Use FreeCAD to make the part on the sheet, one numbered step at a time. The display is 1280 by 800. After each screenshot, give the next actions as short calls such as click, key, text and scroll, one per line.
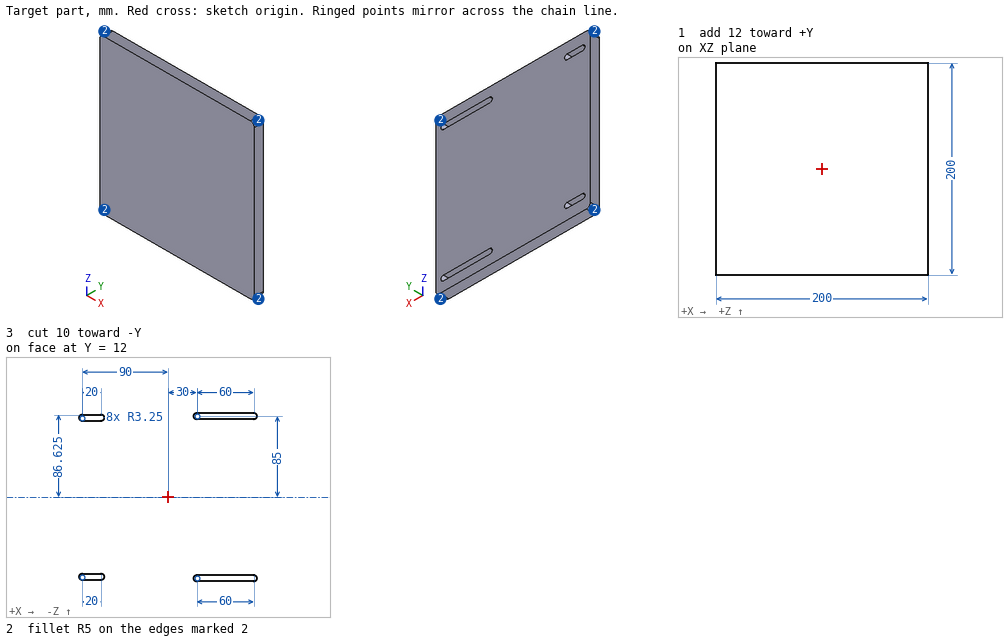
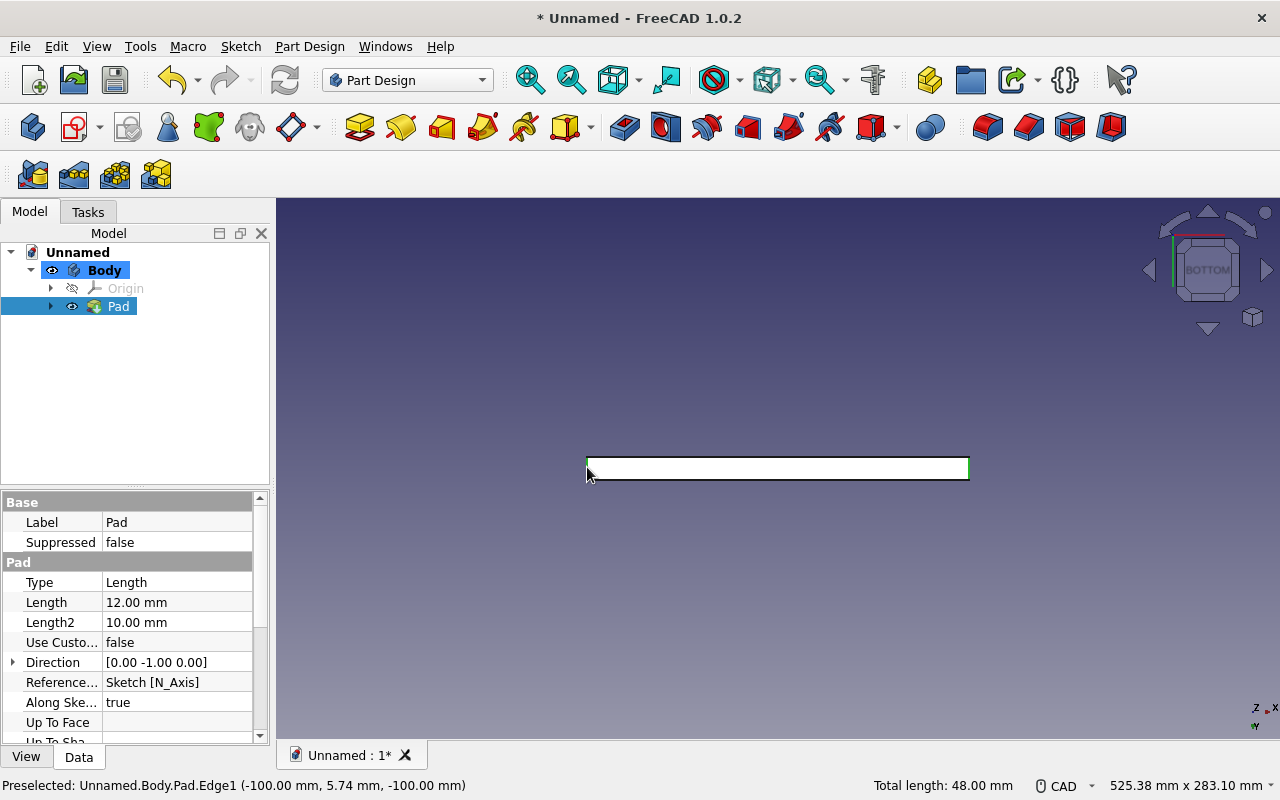
click(988, 128)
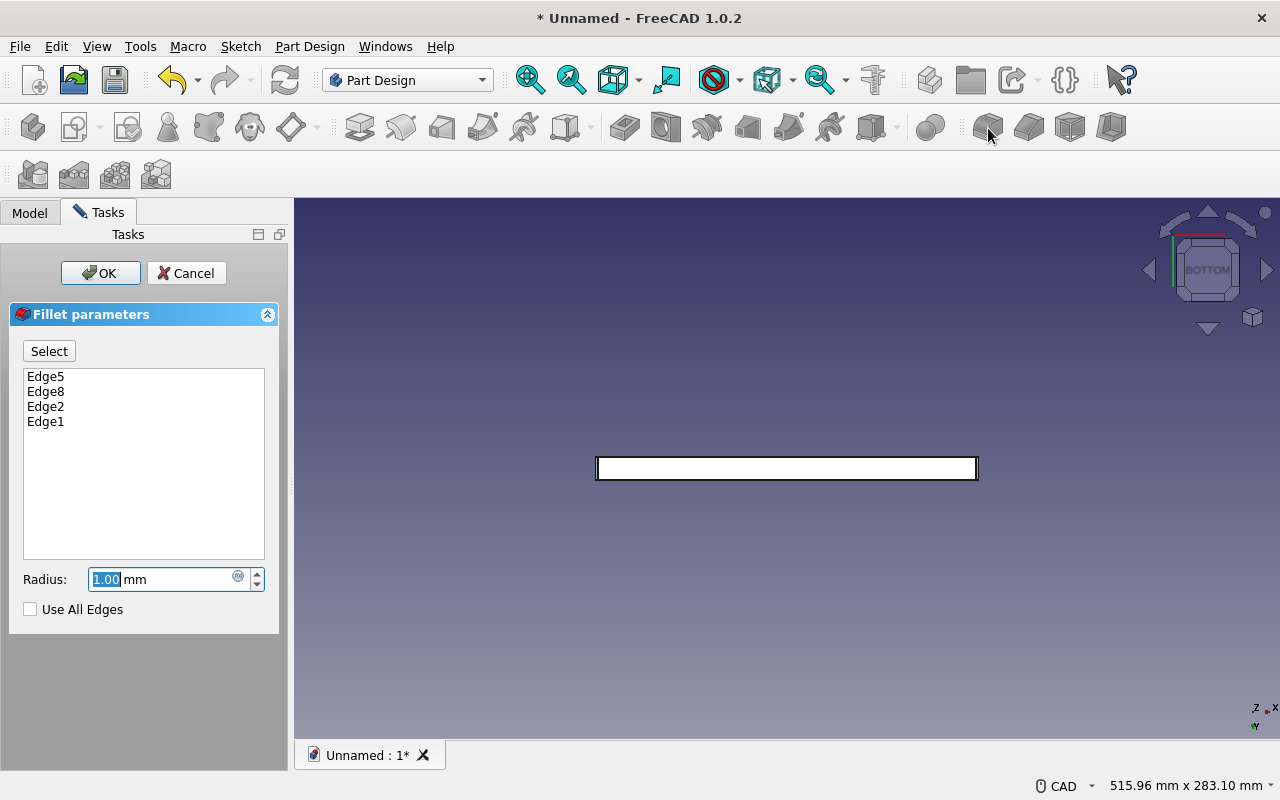
text(5)
key(Tab)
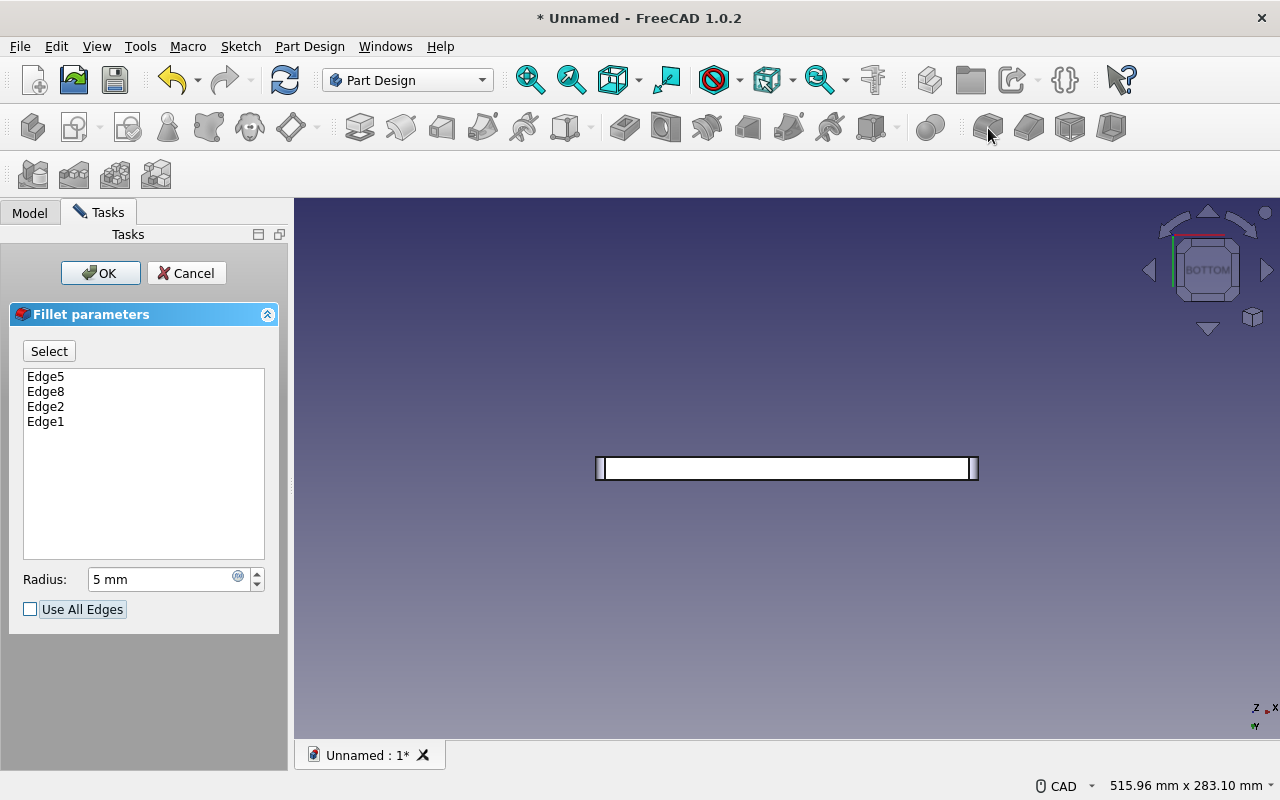
click(101, 273)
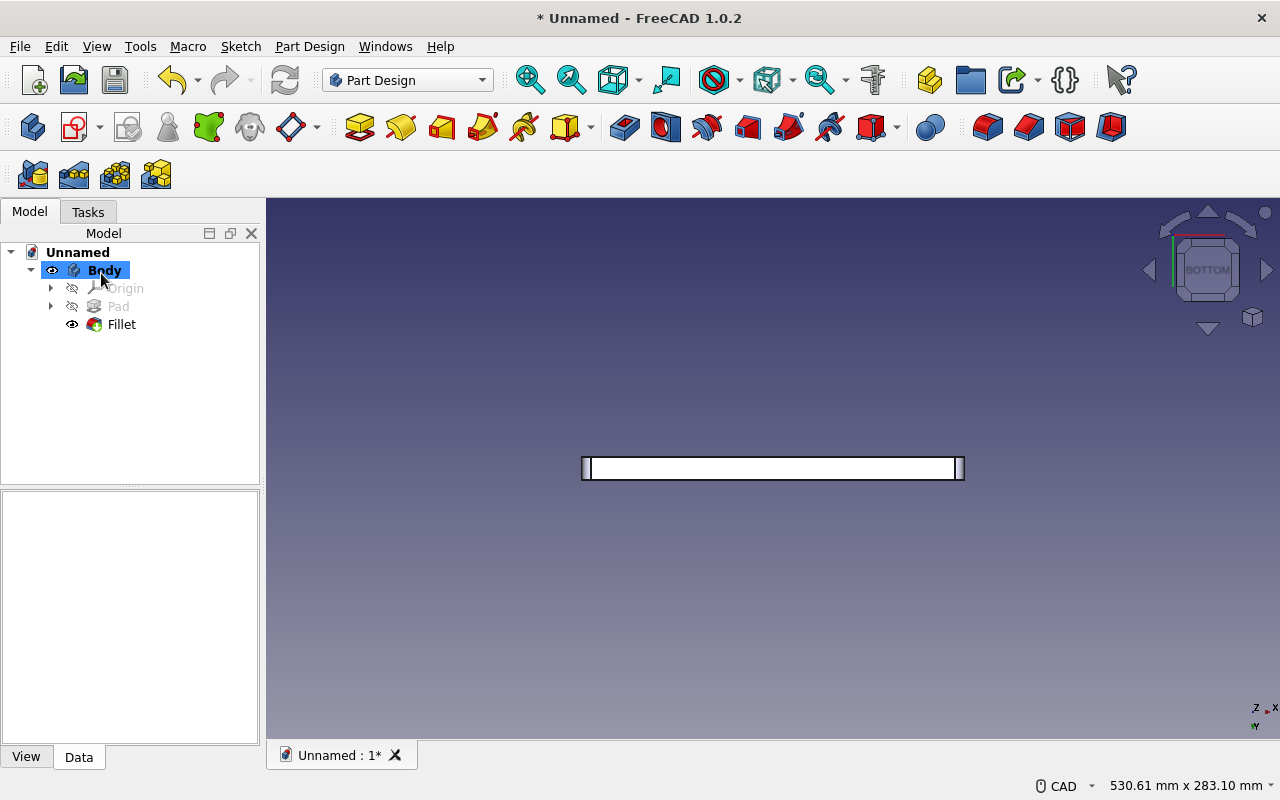
click(531, 80)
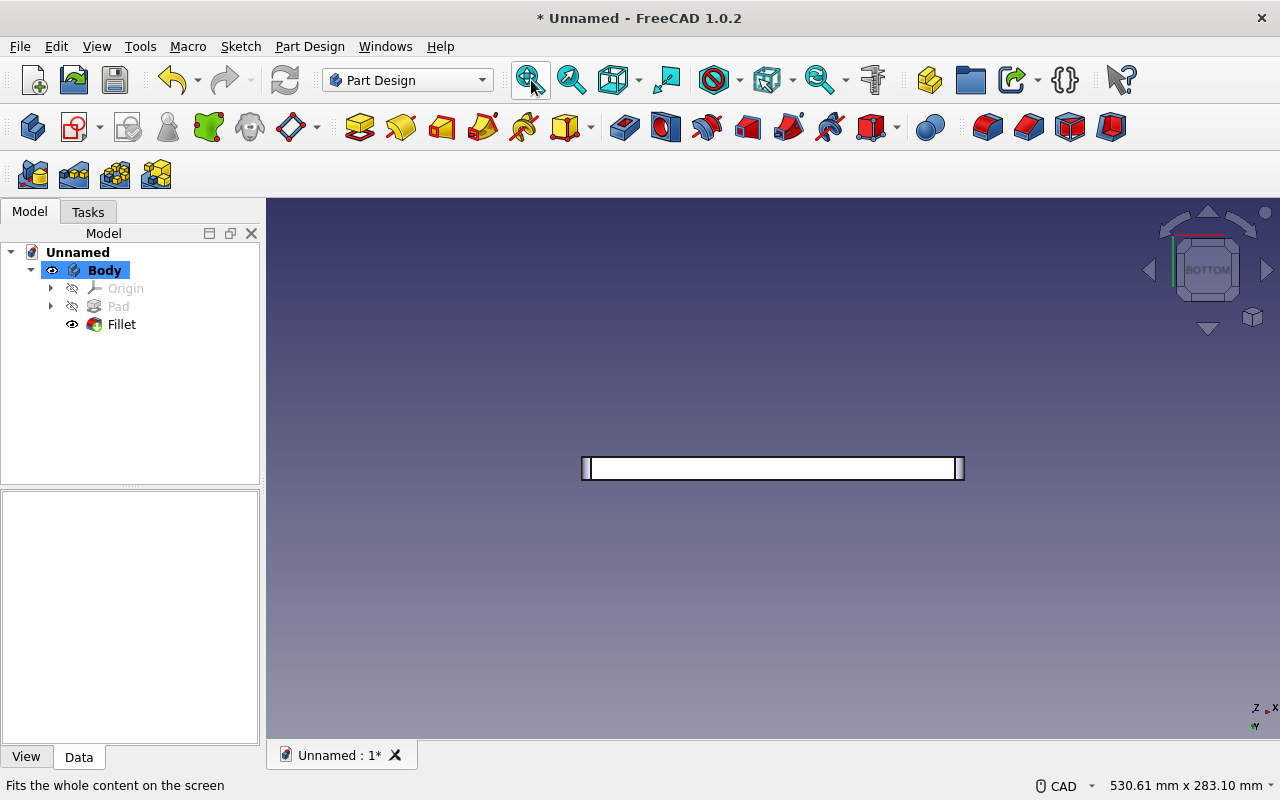
key(4)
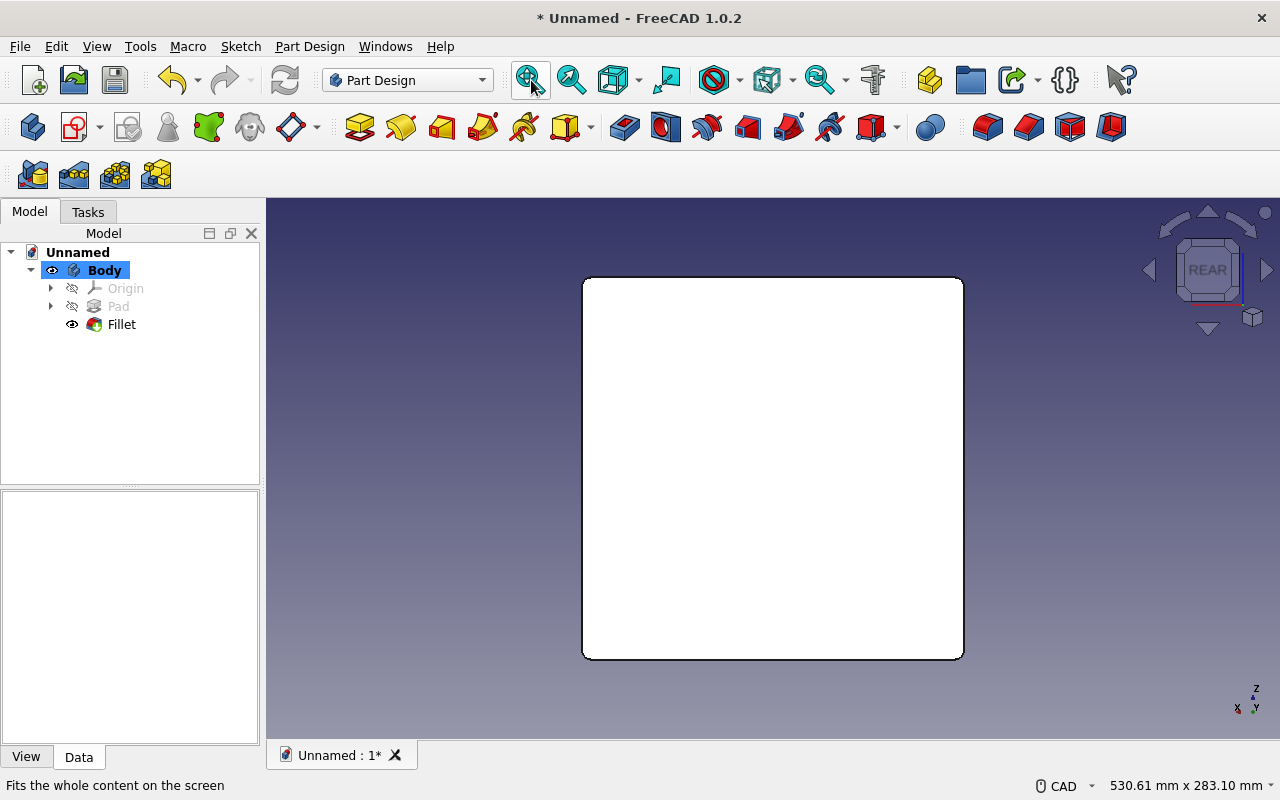
click(773, 467)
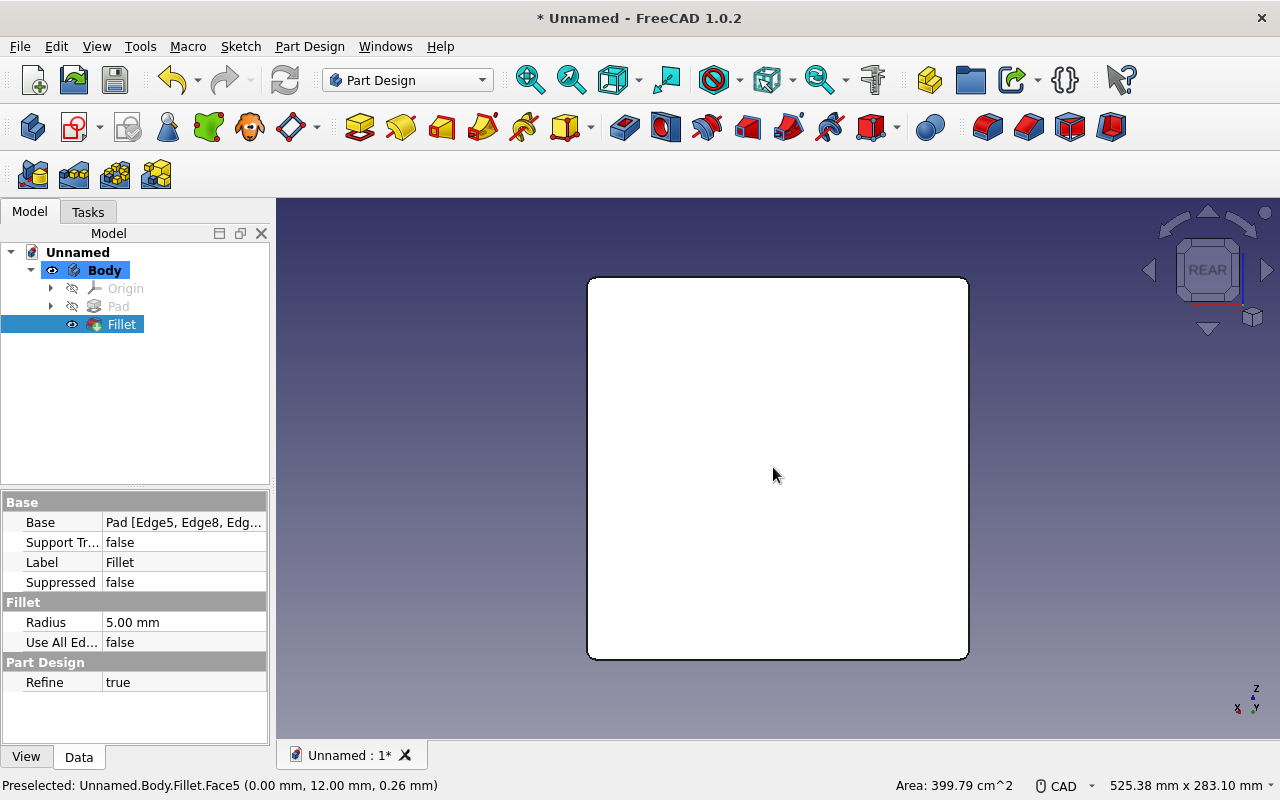
click(74, 128)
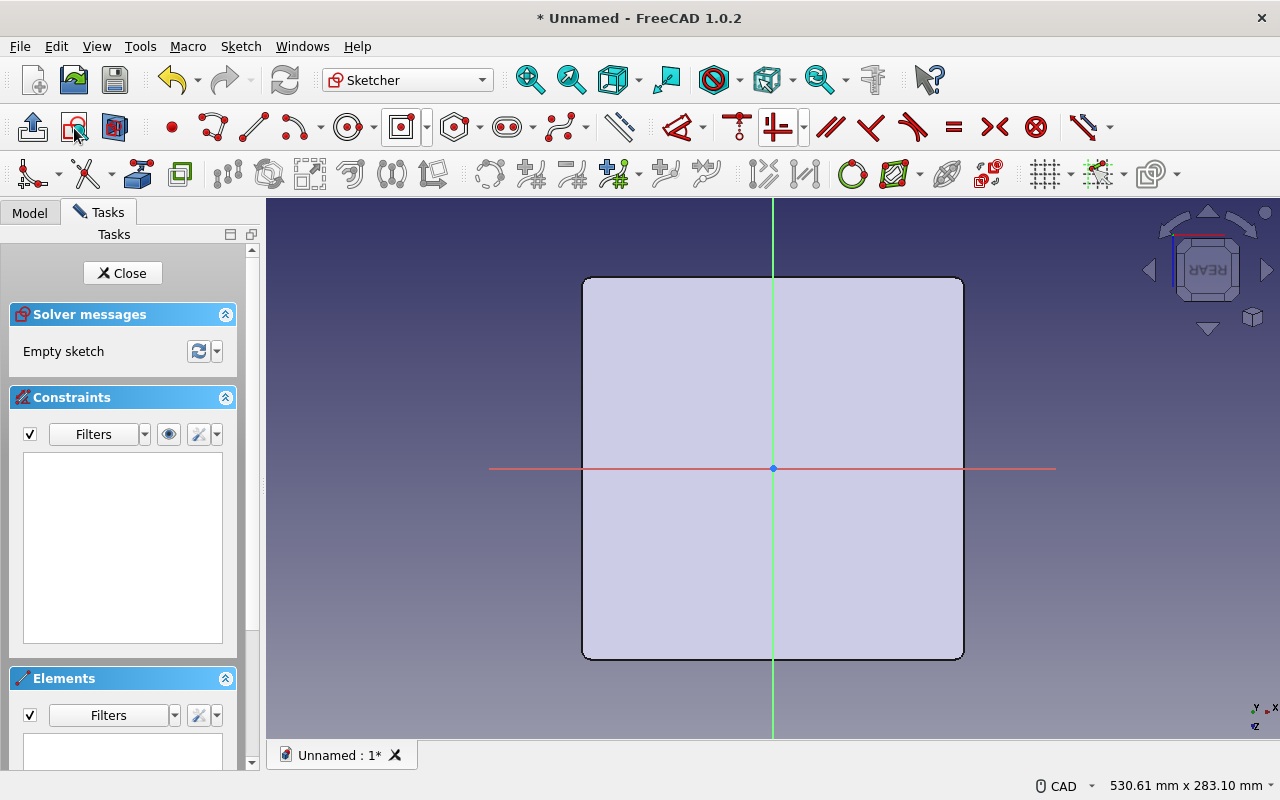
click(506, 128)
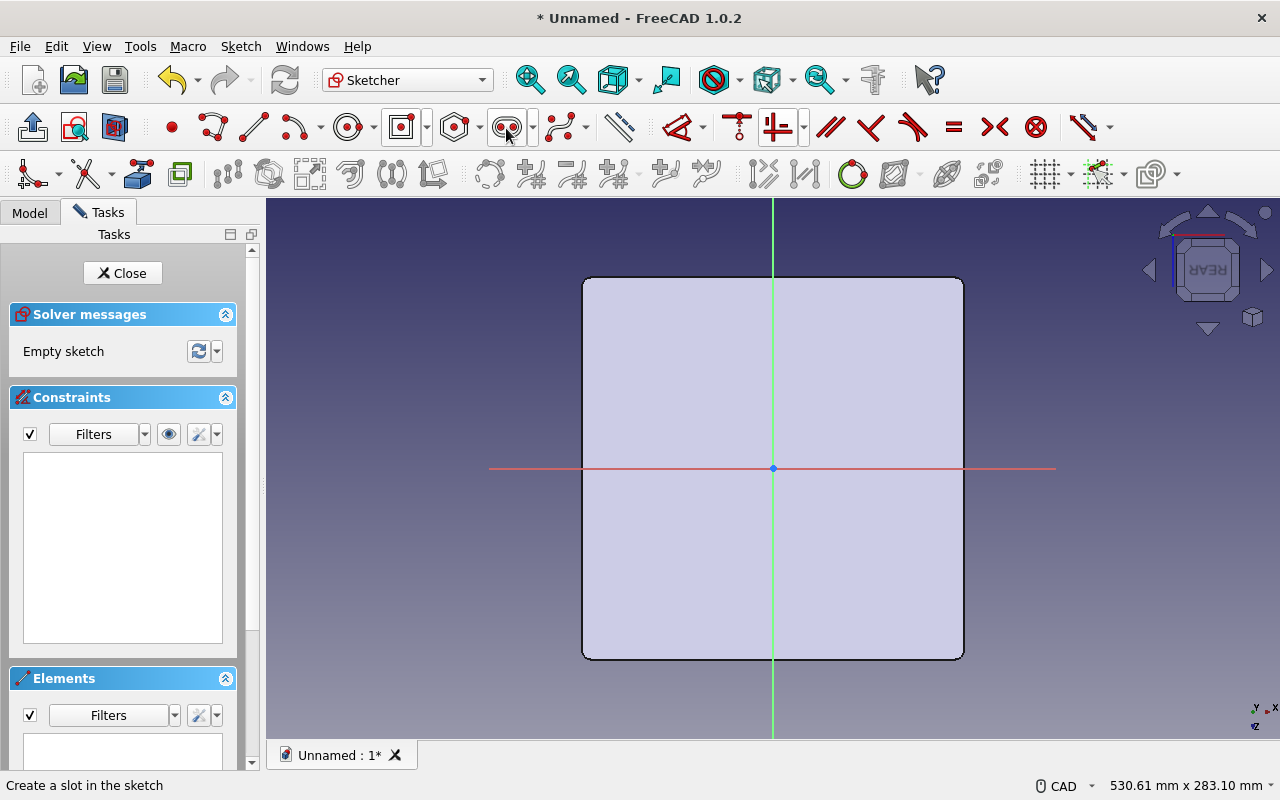
scroll(601, 309, up, 7)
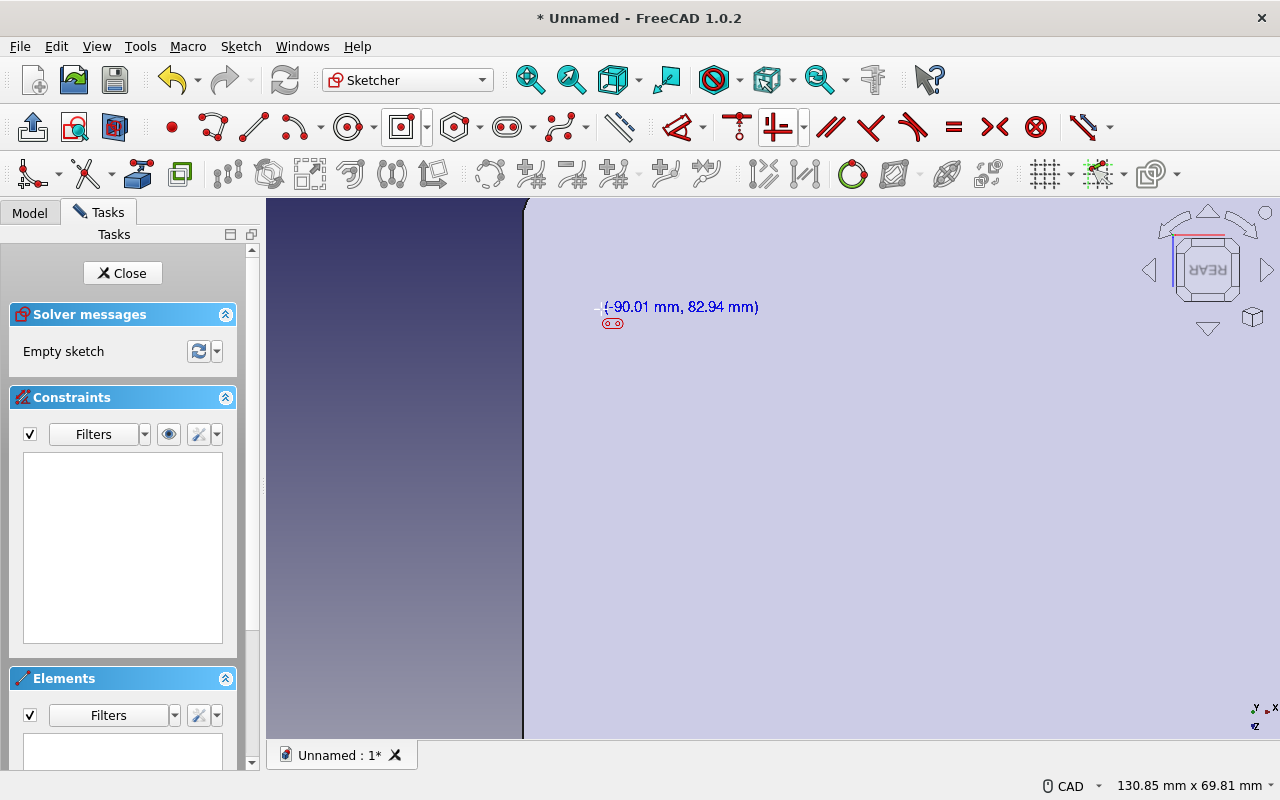
scroll(510, 309, down, 7)